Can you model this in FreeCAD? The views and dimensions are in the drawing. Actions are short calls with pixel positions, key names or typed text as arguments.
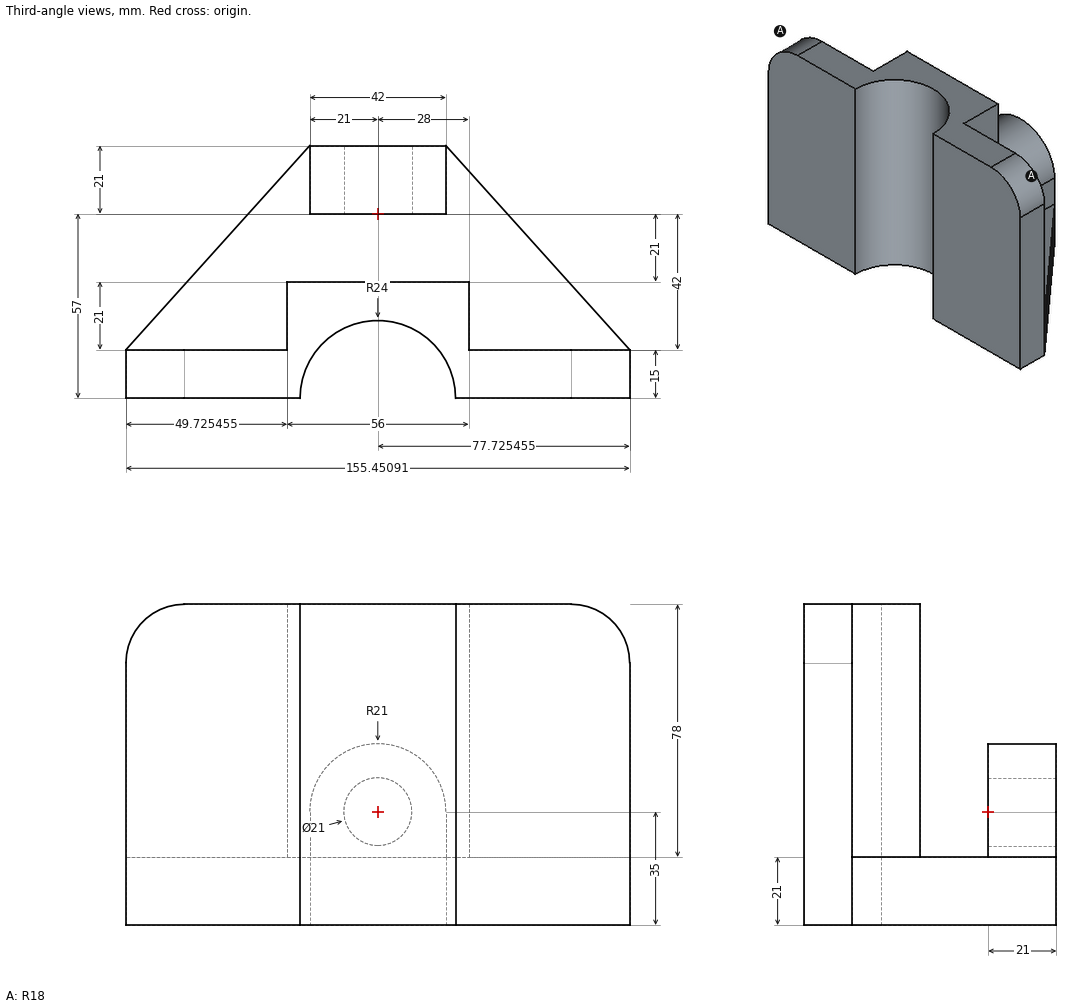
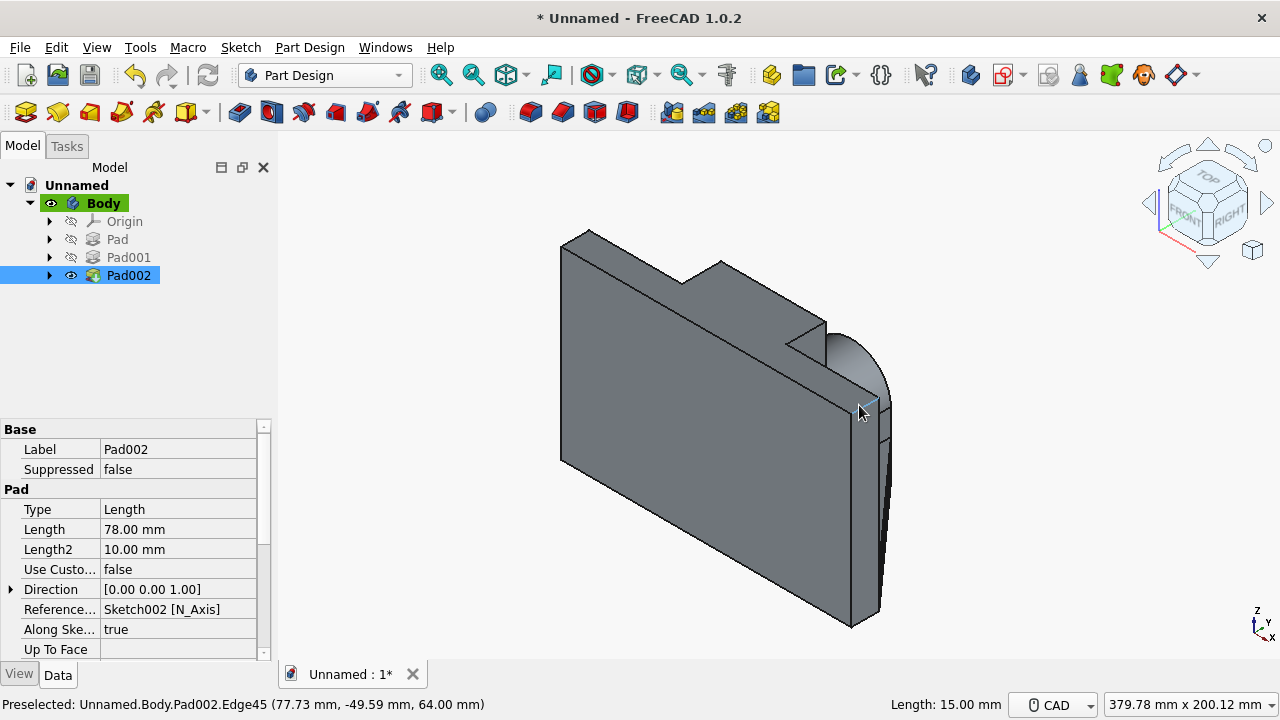
key(2)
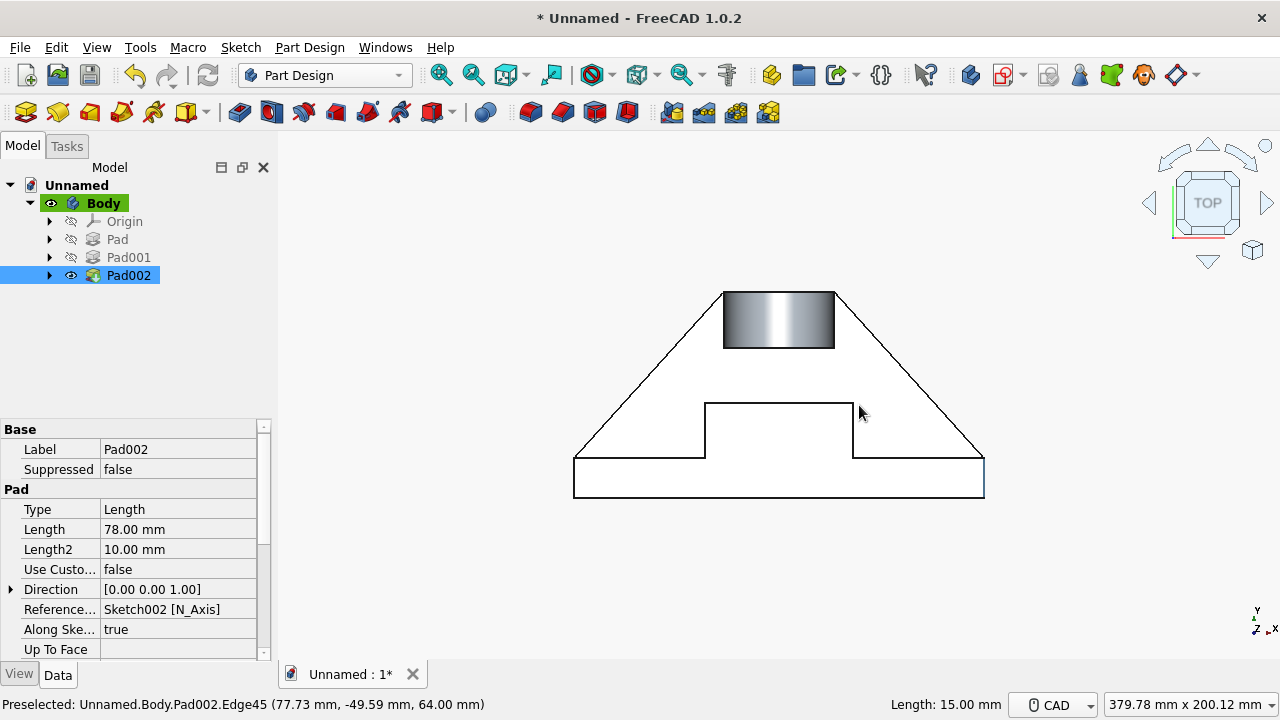
click(442, 76)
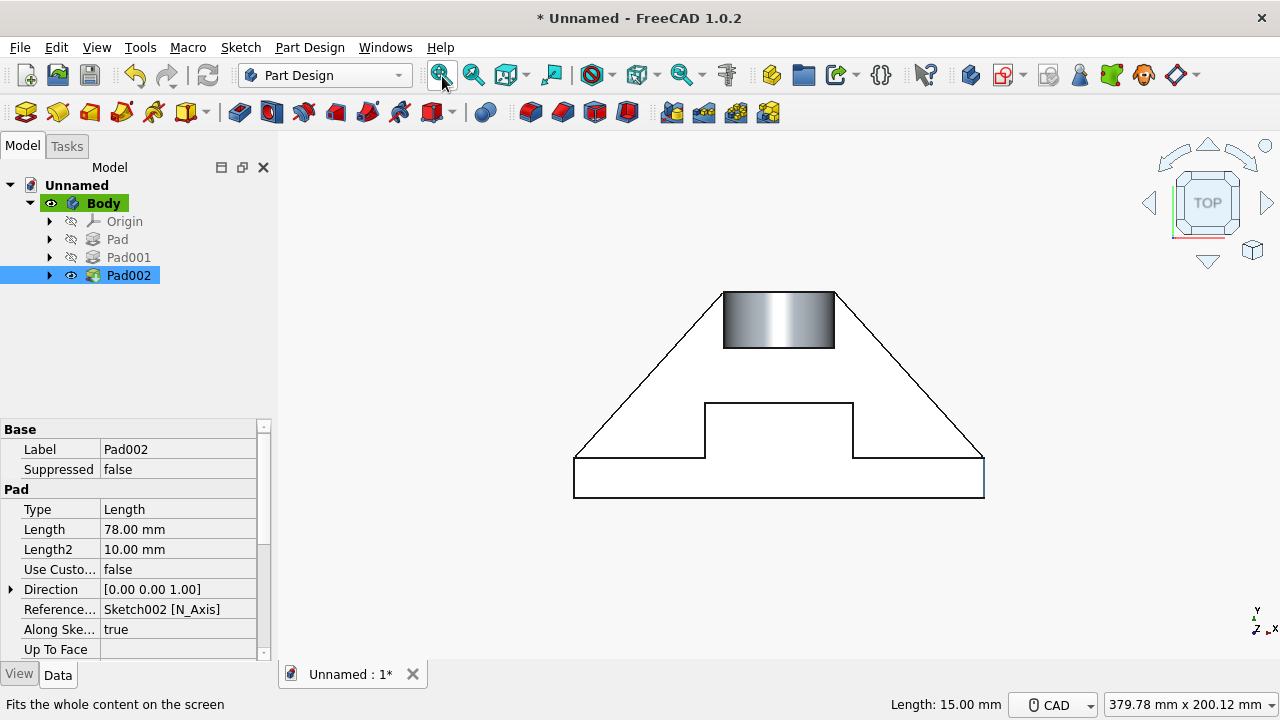
click(574, 477, ctrl)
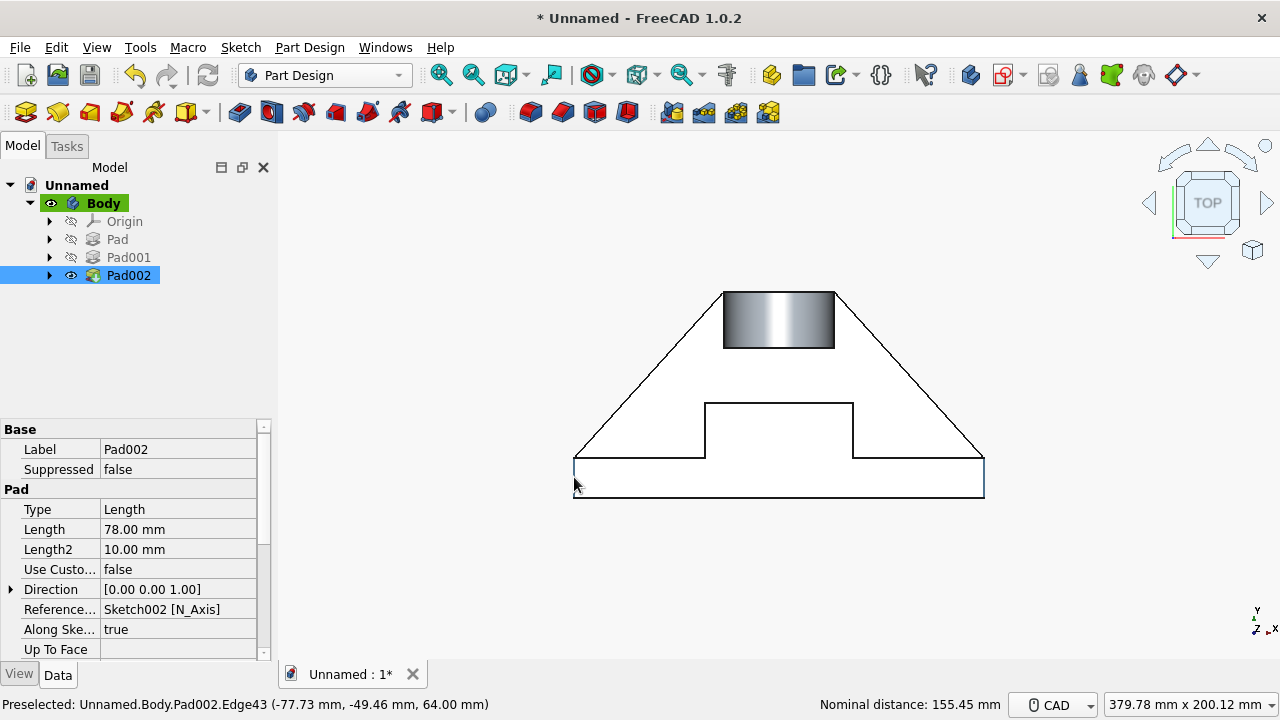
click(532, 112)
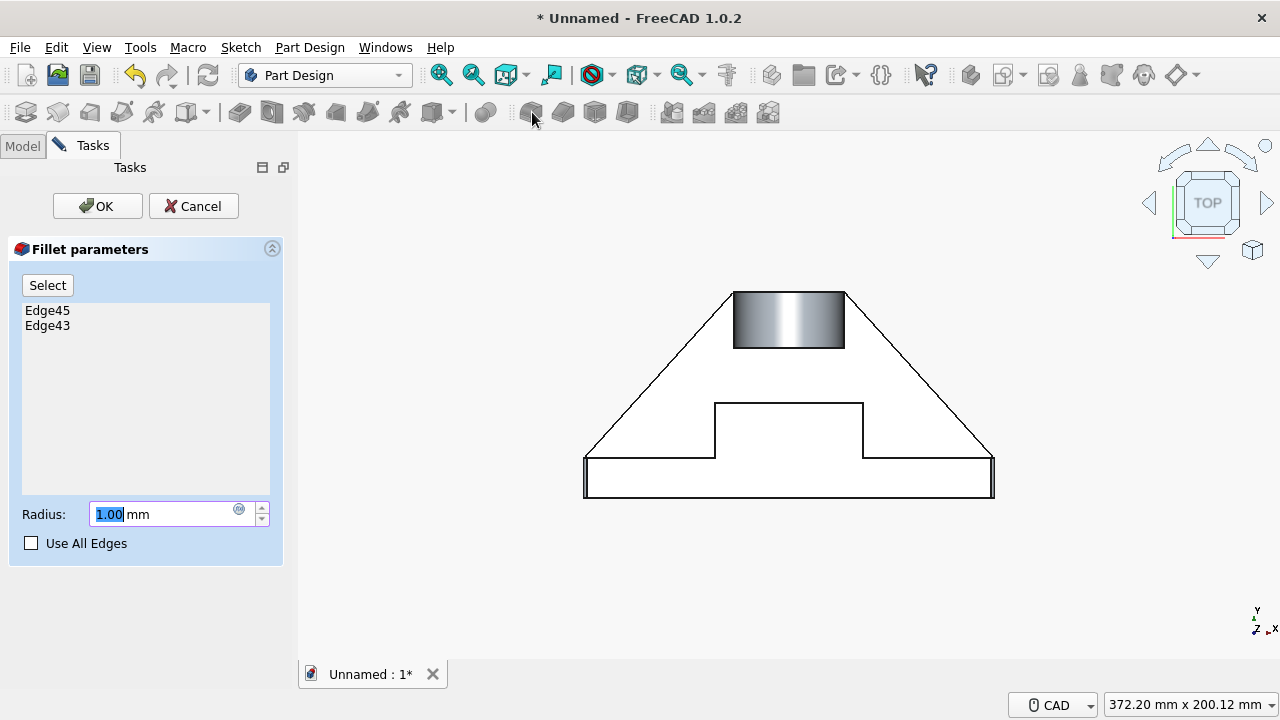
text(18)
key(Tab)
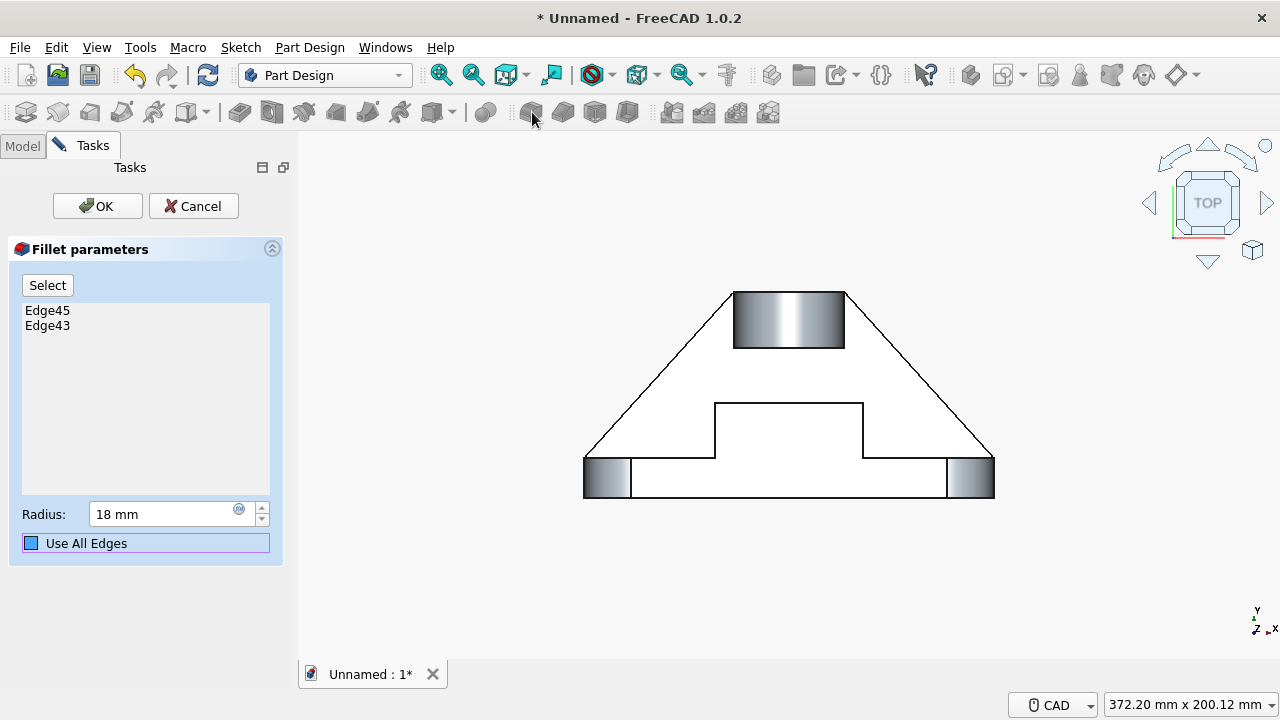
click(98, 206)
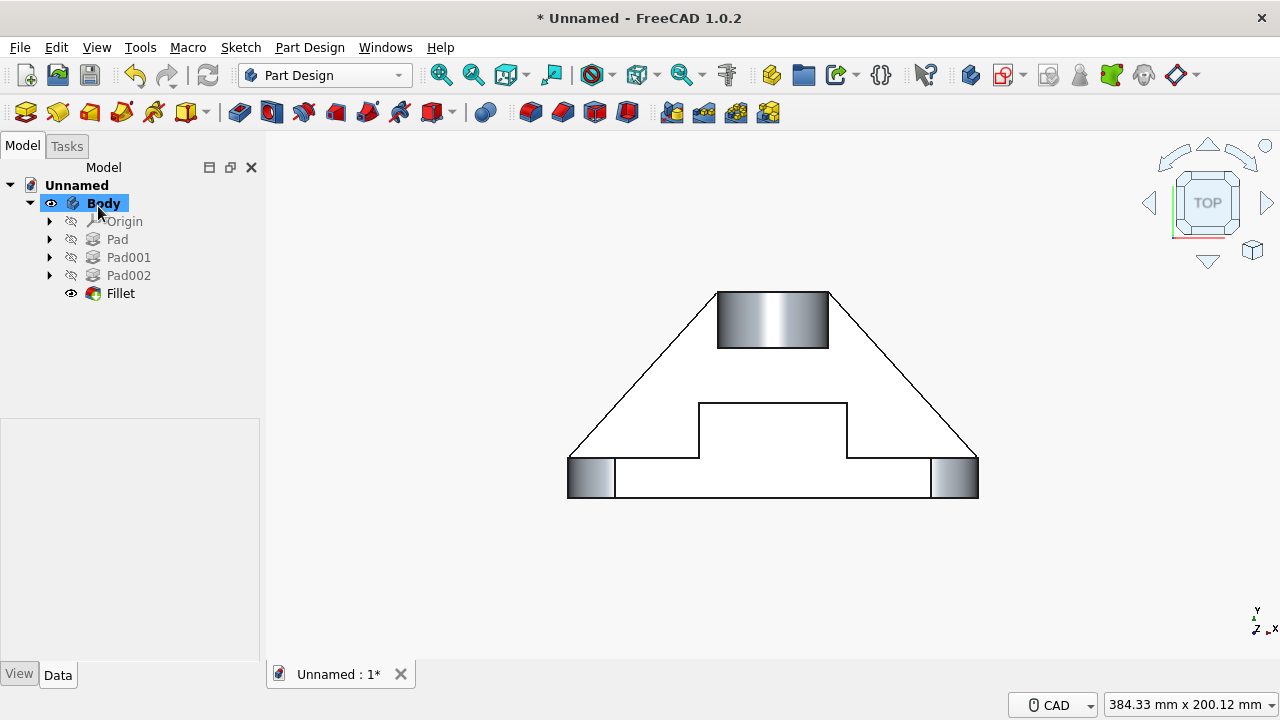
click(442, 76)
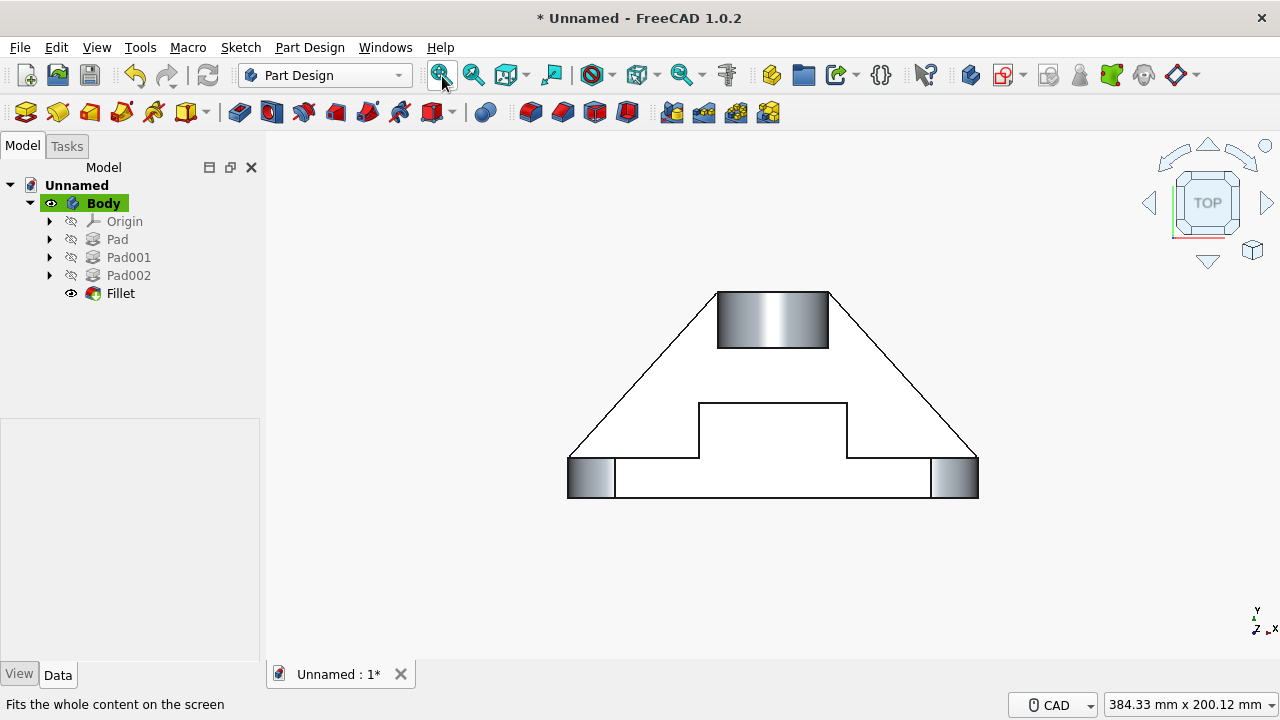
click(773, 449)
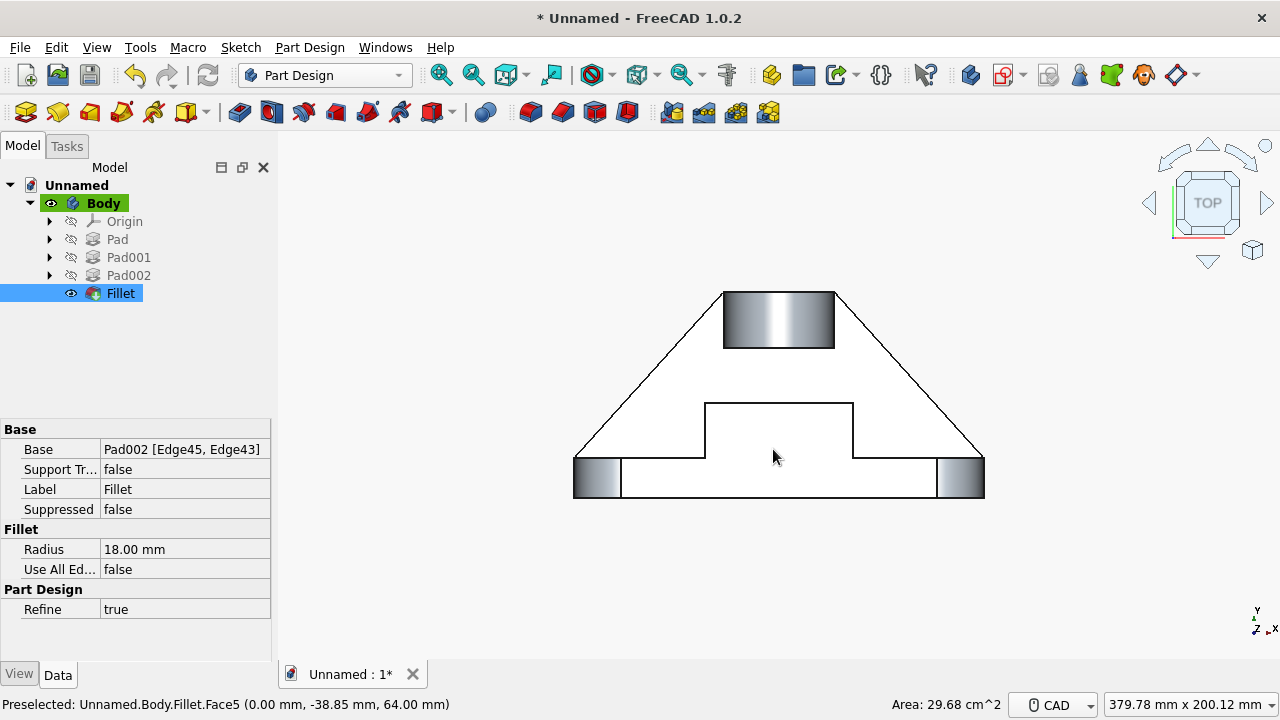
click(1004, 76)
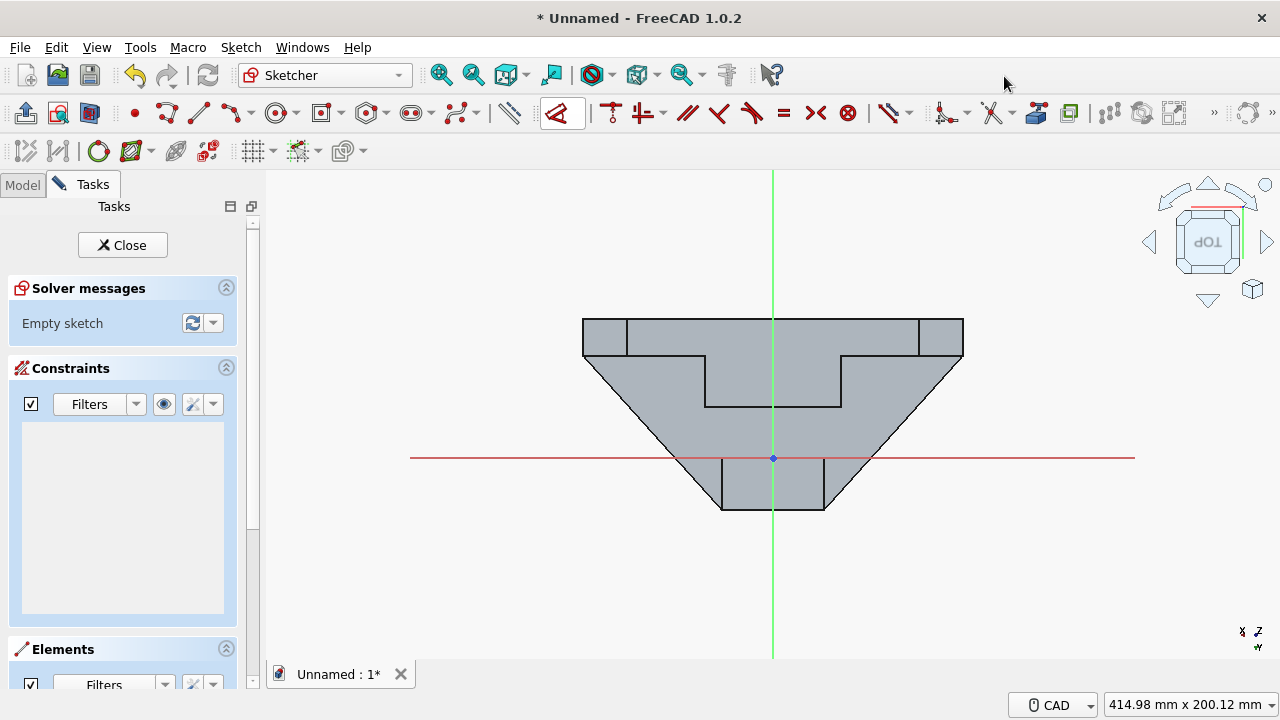
scroll(829, 368, up, 4)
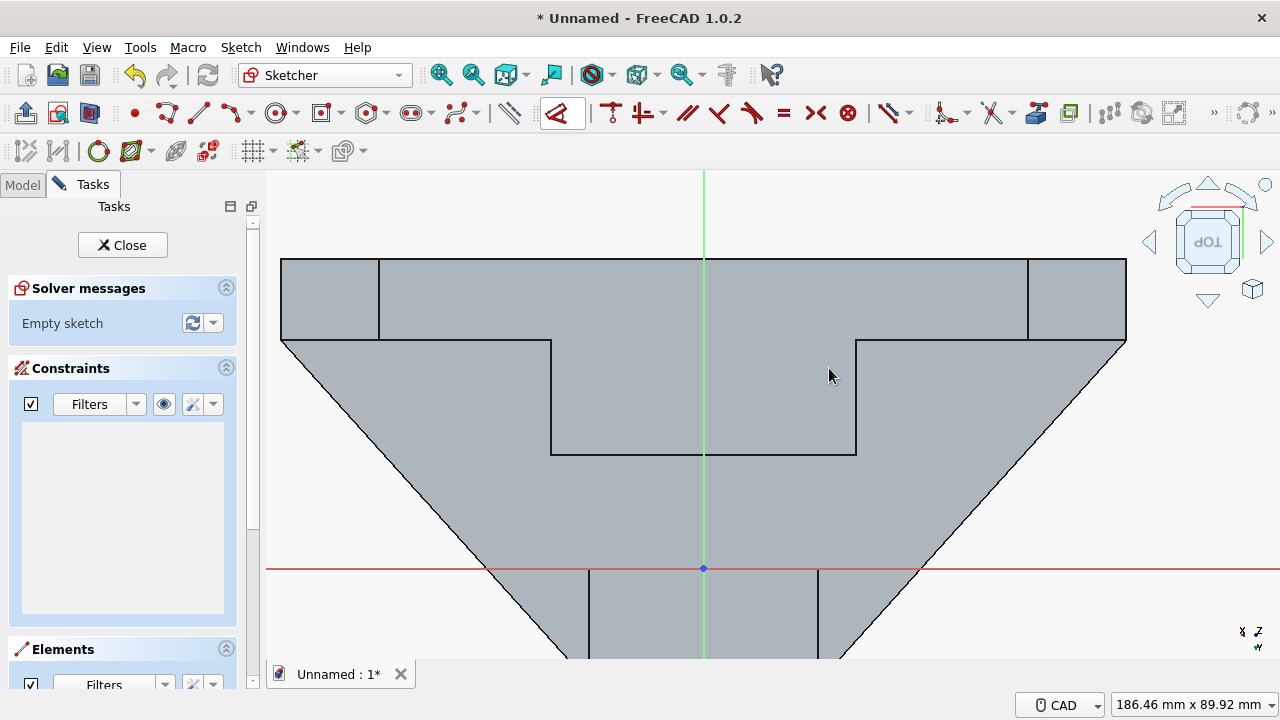
key(g)
key(l)